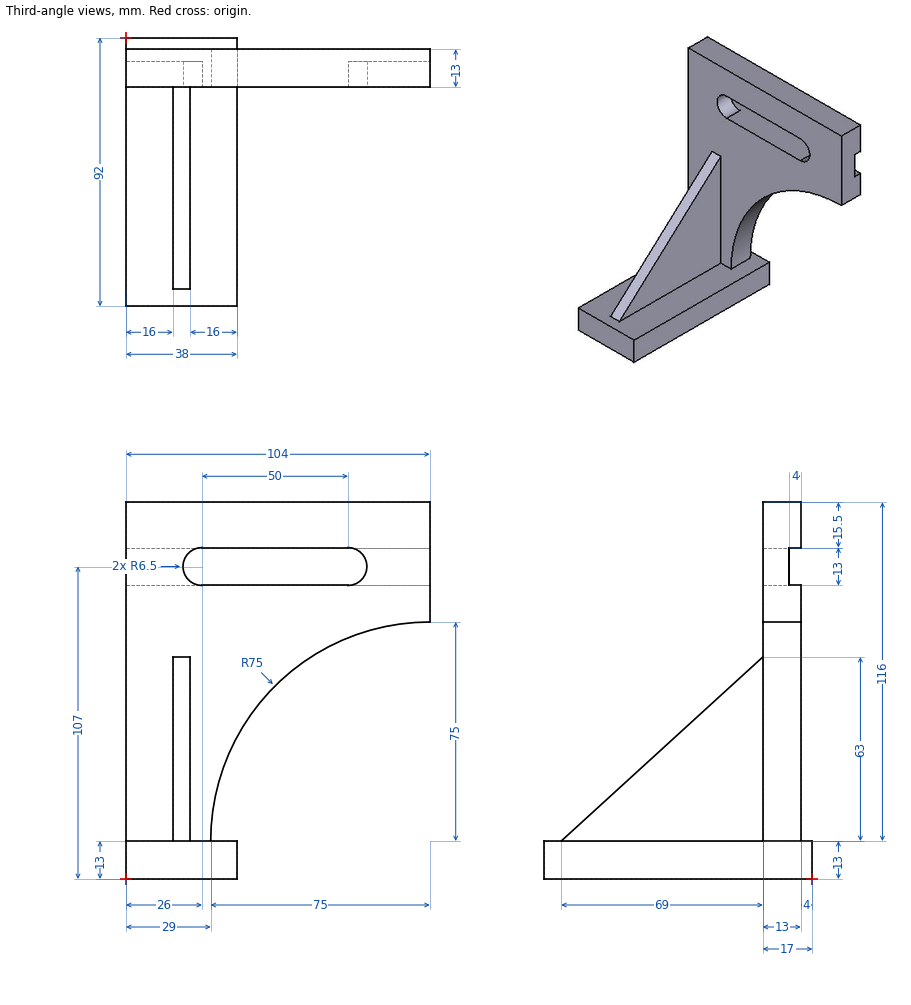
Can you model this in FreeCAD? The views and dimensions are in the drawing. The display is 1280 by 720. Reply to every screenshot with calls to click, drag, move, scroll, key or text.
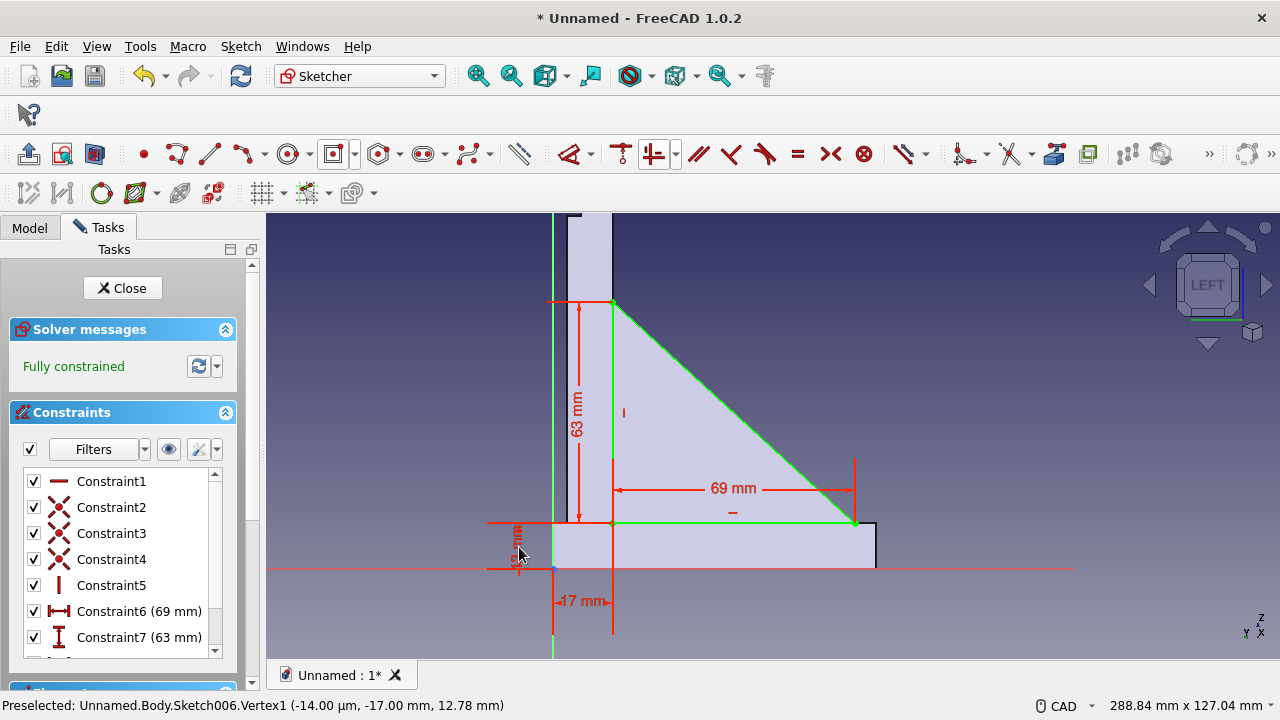
click(123, 288)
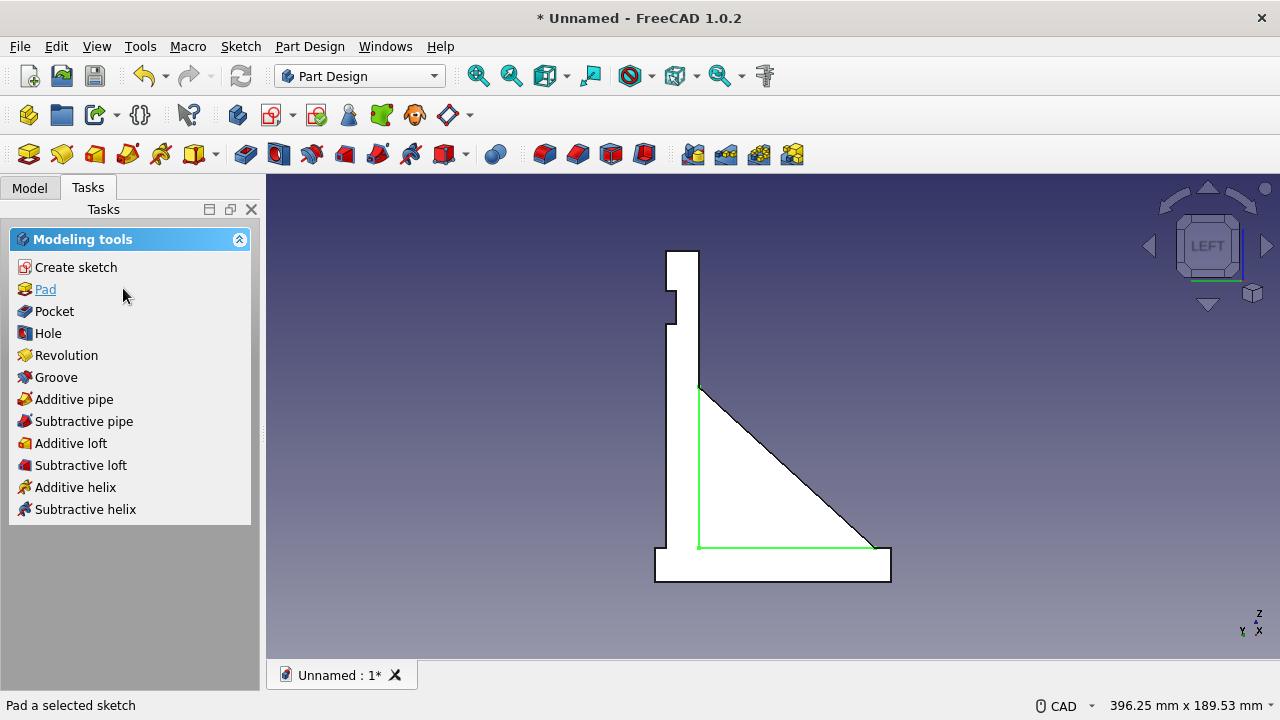
click(246, 154)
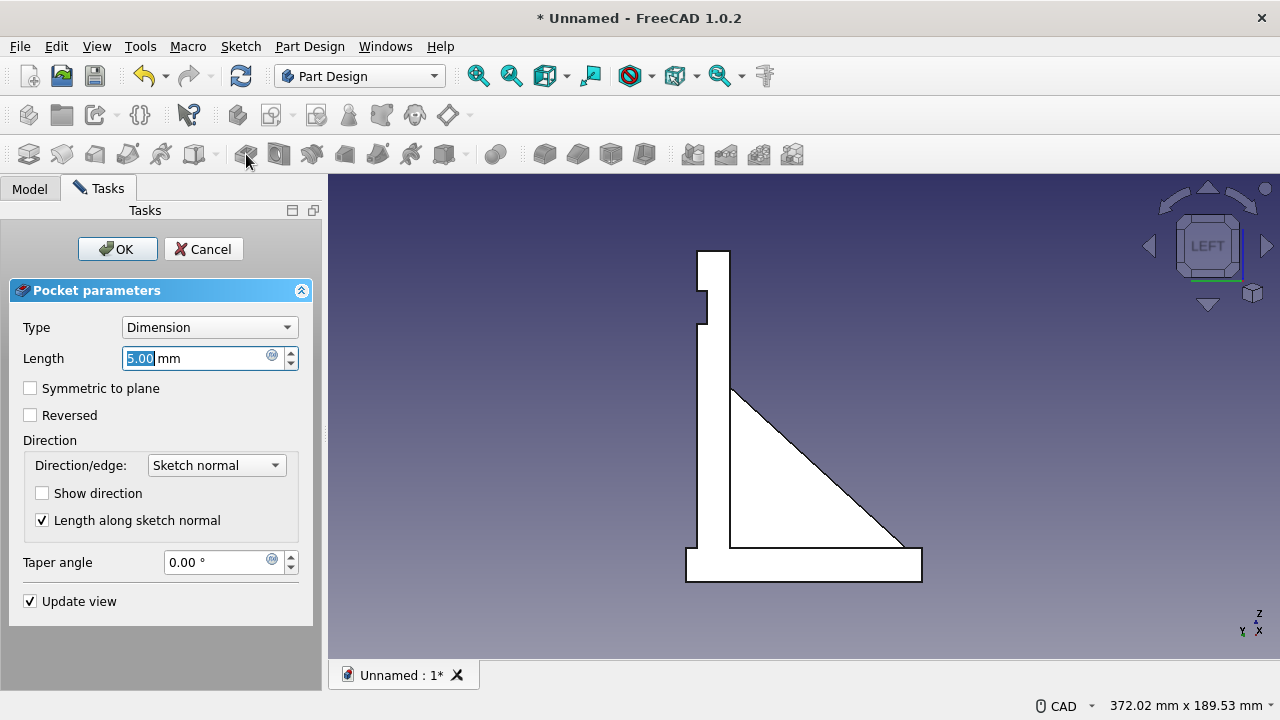
text(16)
key(Tab)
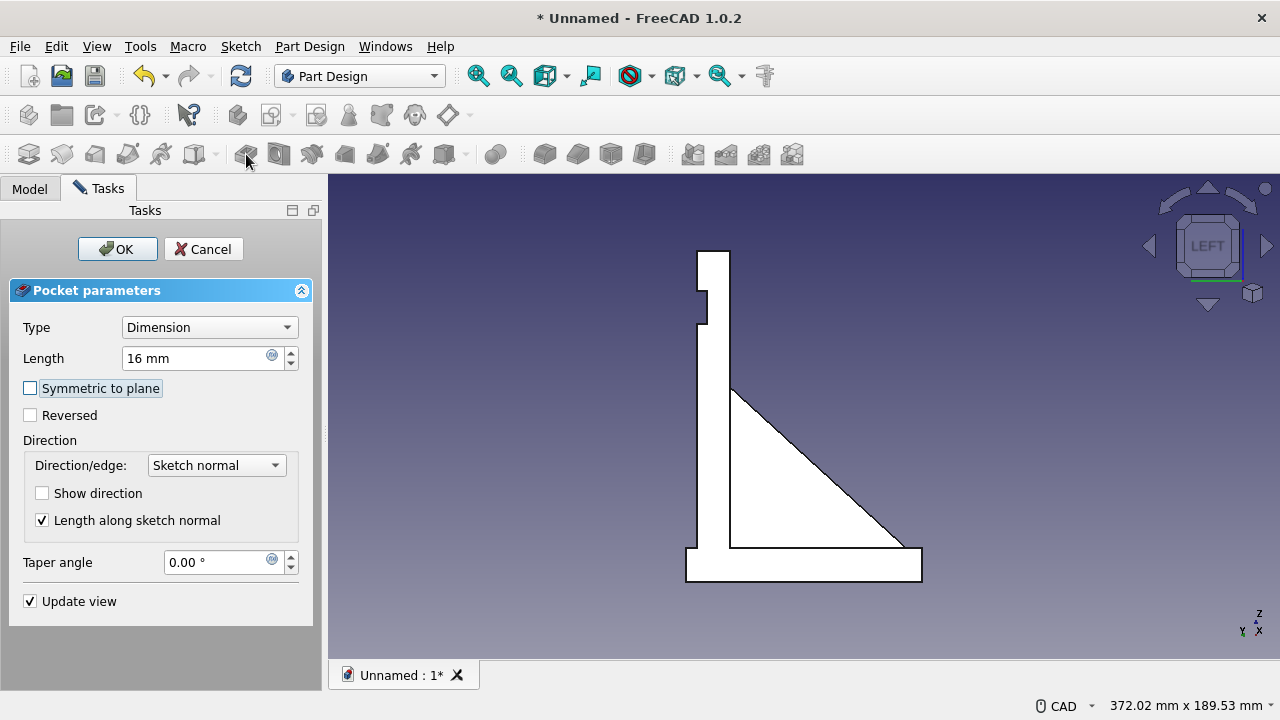
click(118, 249)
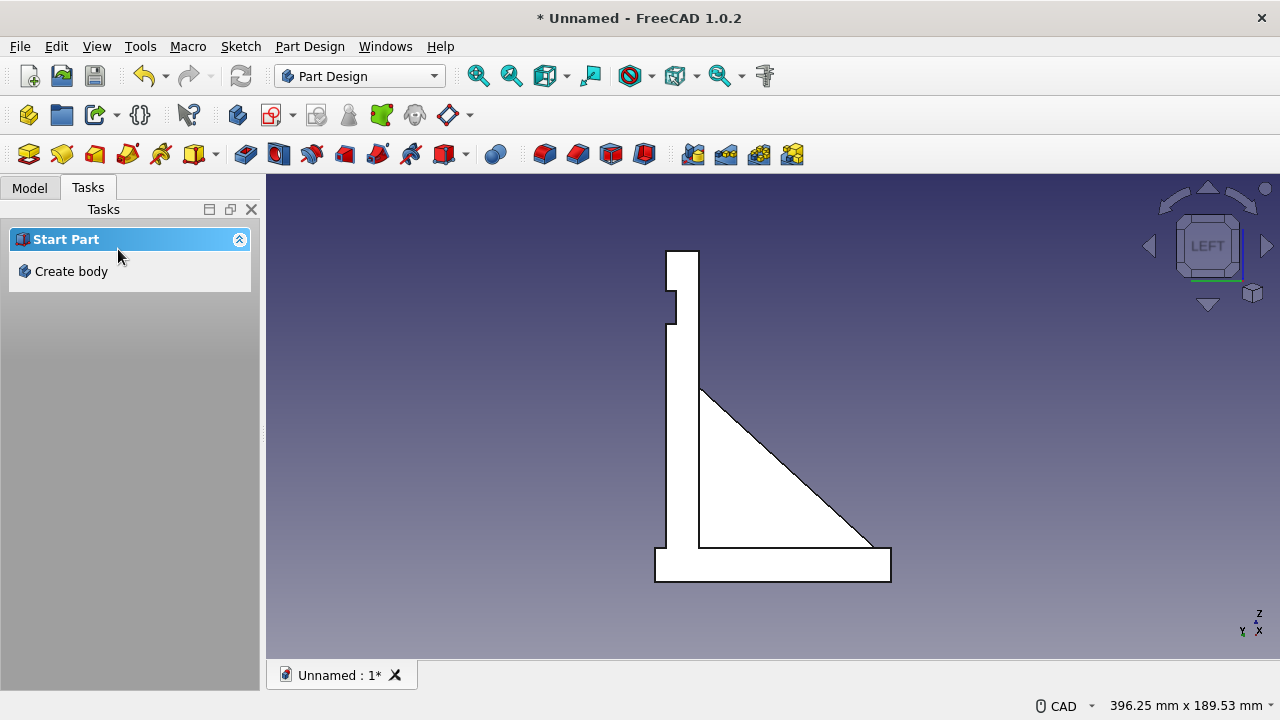
key(0)